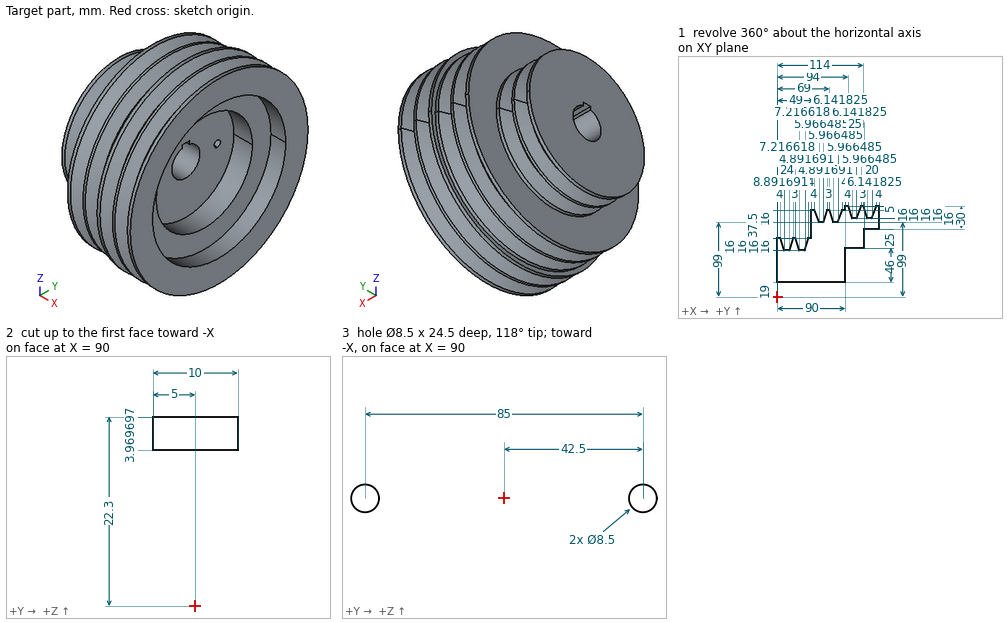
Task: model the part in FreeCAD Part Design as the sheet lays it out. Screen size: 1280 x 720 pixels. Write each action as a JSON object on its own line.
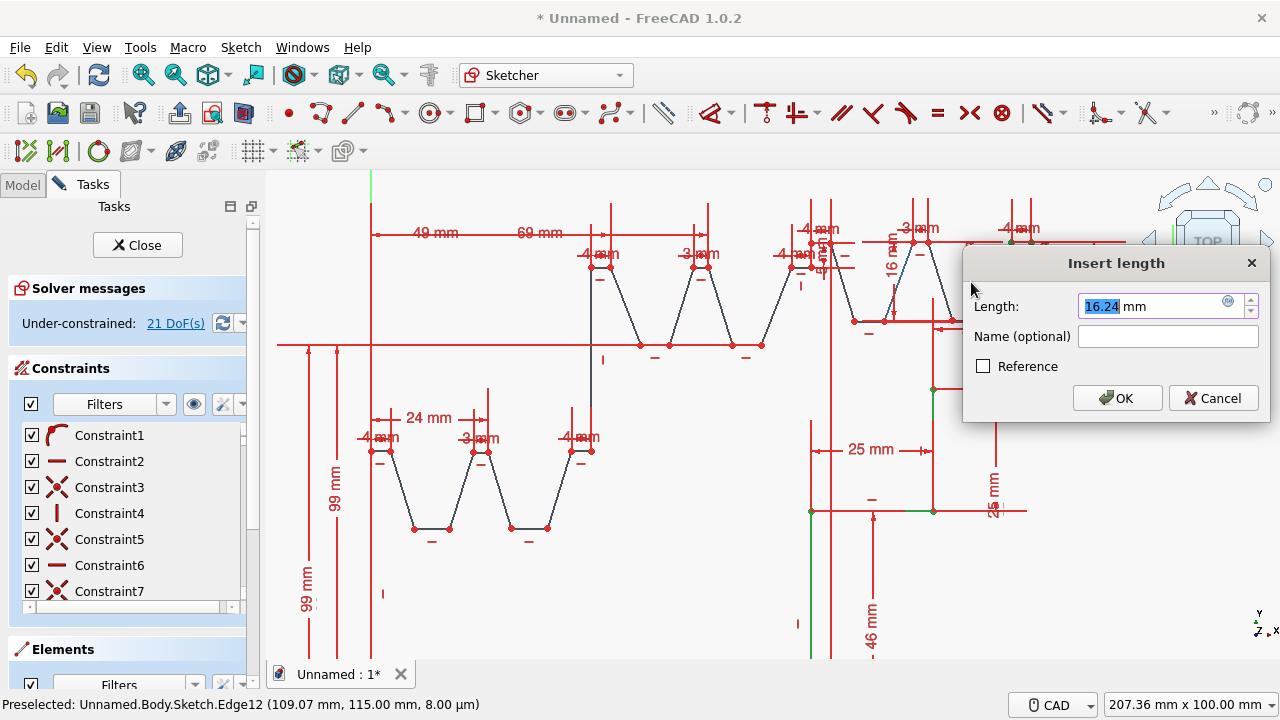
{"action": "type", "text": "16"}
{"action": "key", "text": "Return"}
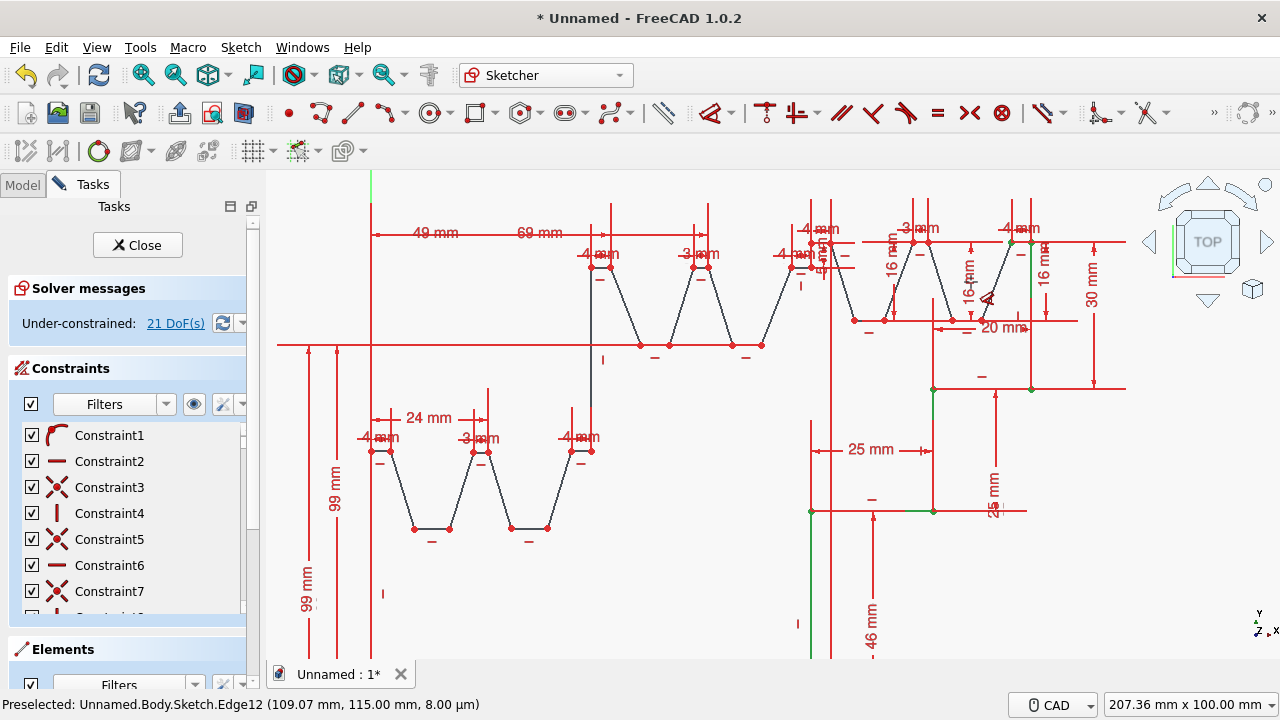
{"action": "left_click", "coordinate": [847, 297]}
{"action": "left_click", "coordinate": [797, 300]}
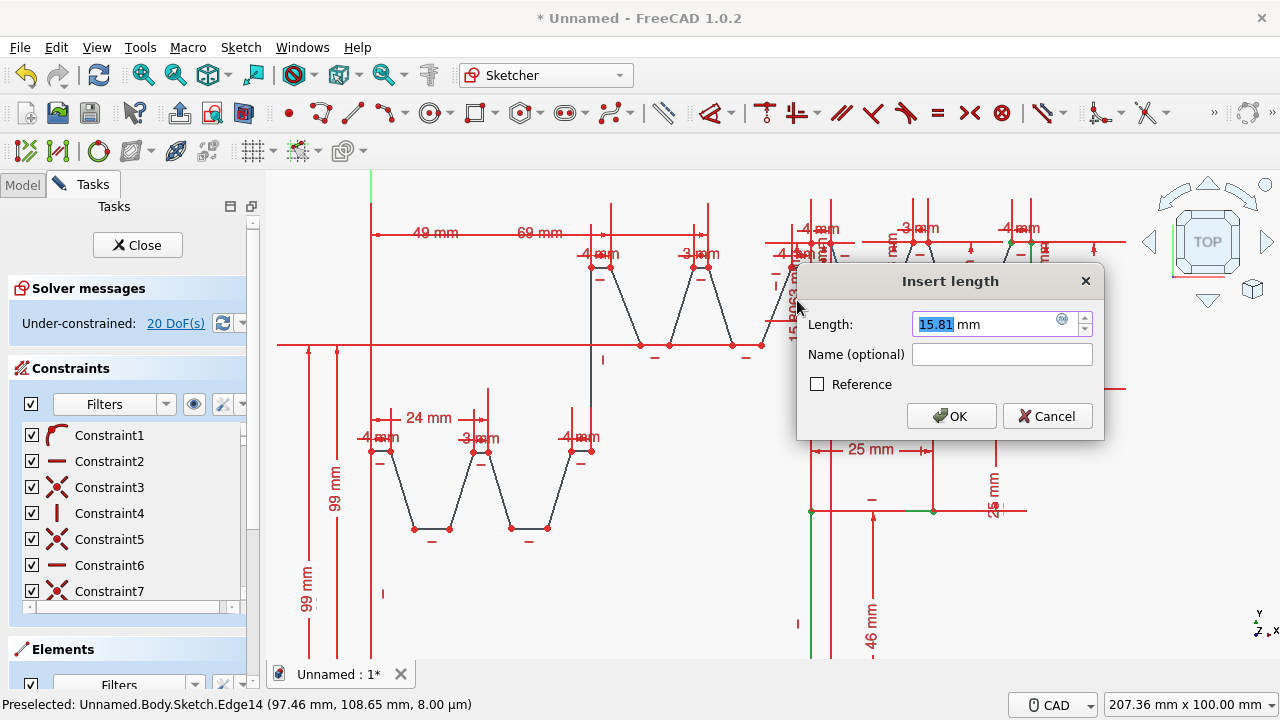
{"action": "type", "text": "16"}
{"action": "key", "text": "Return"}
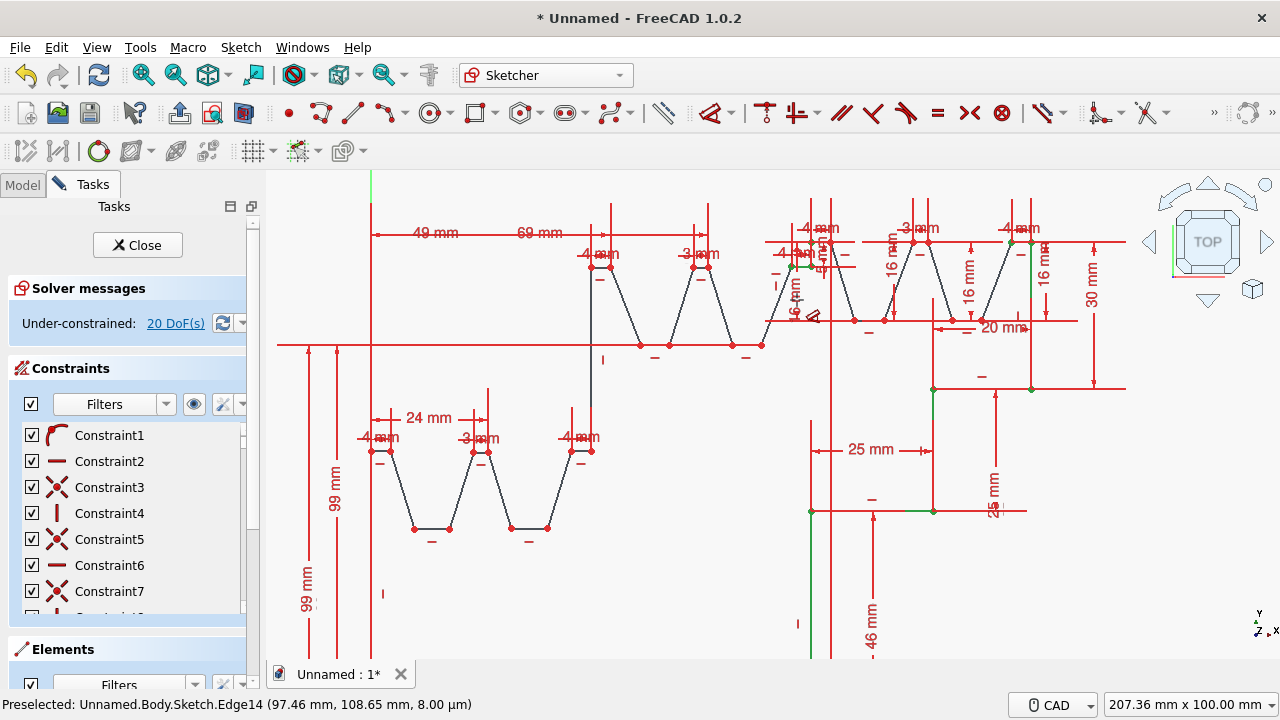
{"action": "left_click", "coordinate": [725, 322]}
{"action": "left_click", "coordinate": [767, 279]}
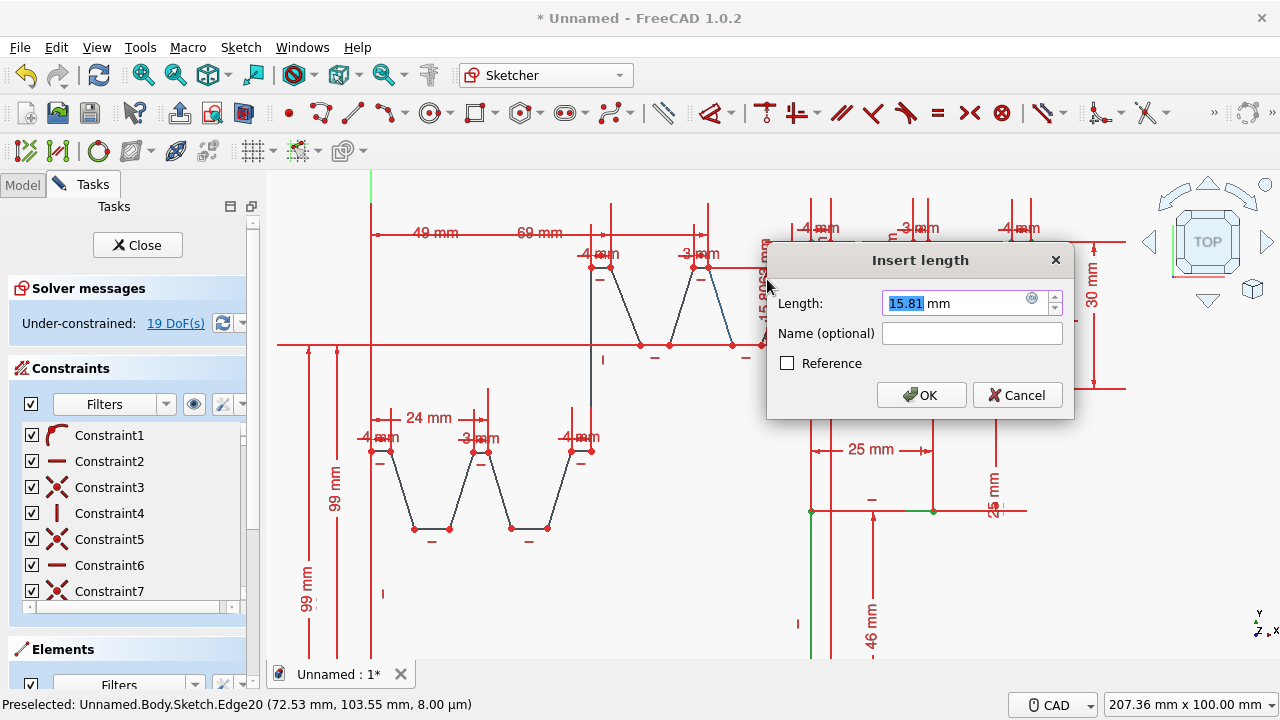
{"action": "type", "text": "16"}
{"action": "key", "text": "Return"}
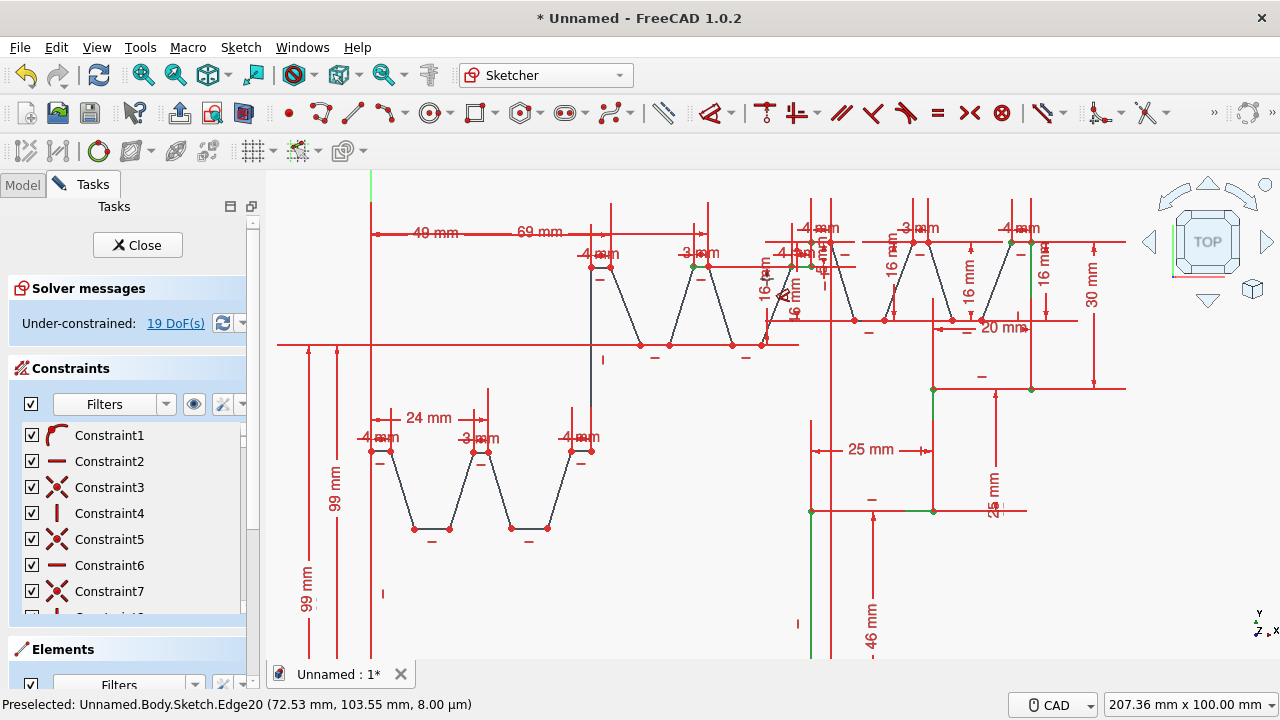
{"action": "left_click", "coordinate": [632, 322]}
{"action": "left_click", "coordinate": [577, 306]}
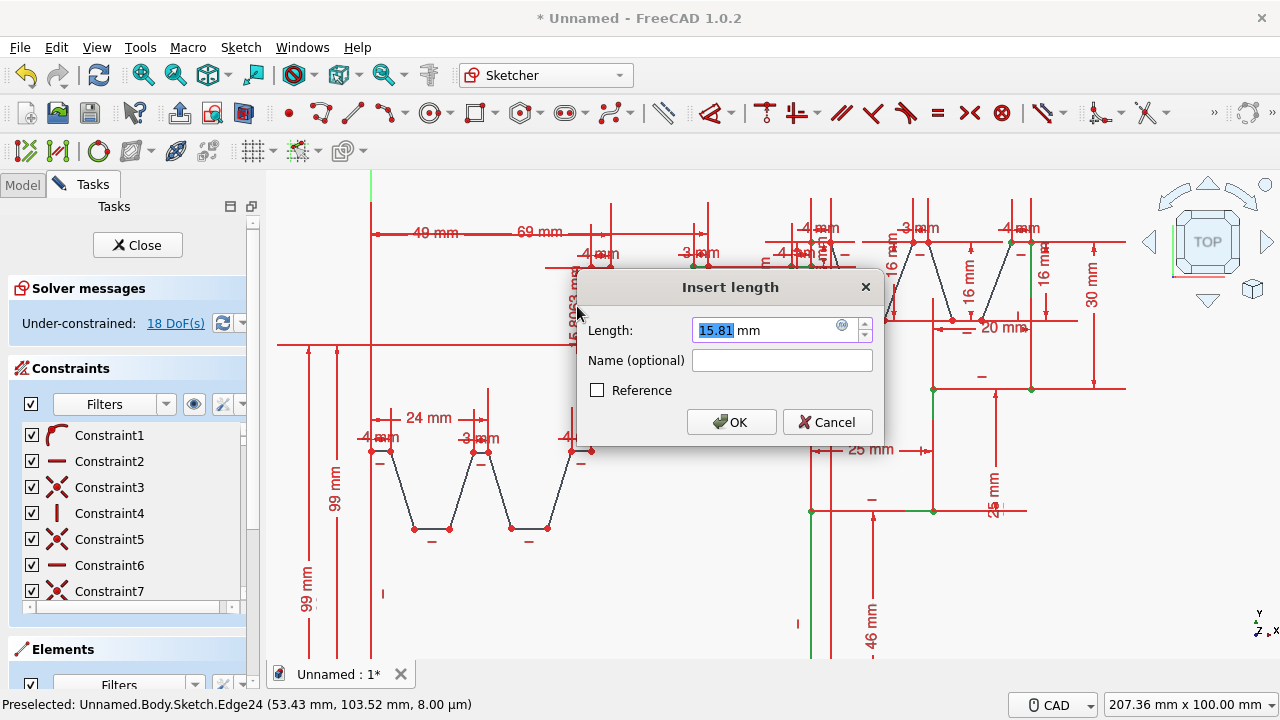
{"action": "type", "text": "16"}
{"action": "key", "text": "Return"}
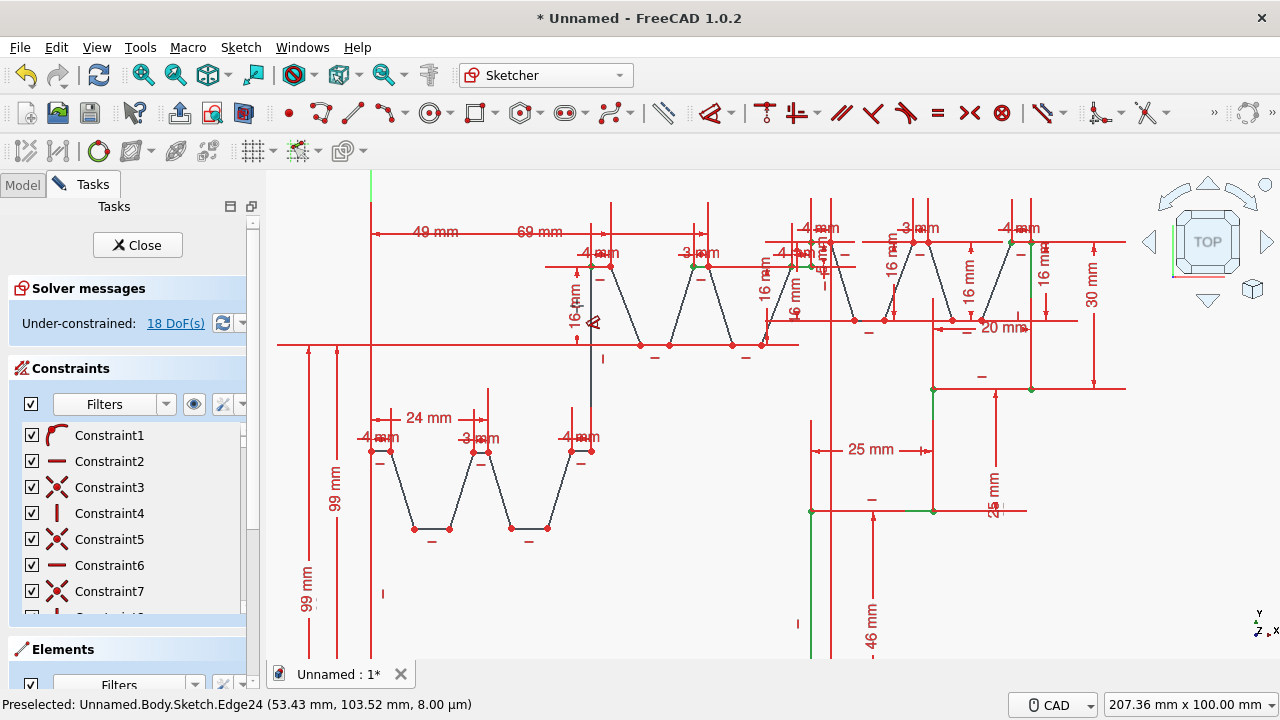
{"action": "left_click", "coordinate": [564, 474]}
{"action": "left_click", "coordinate": [514, 490]}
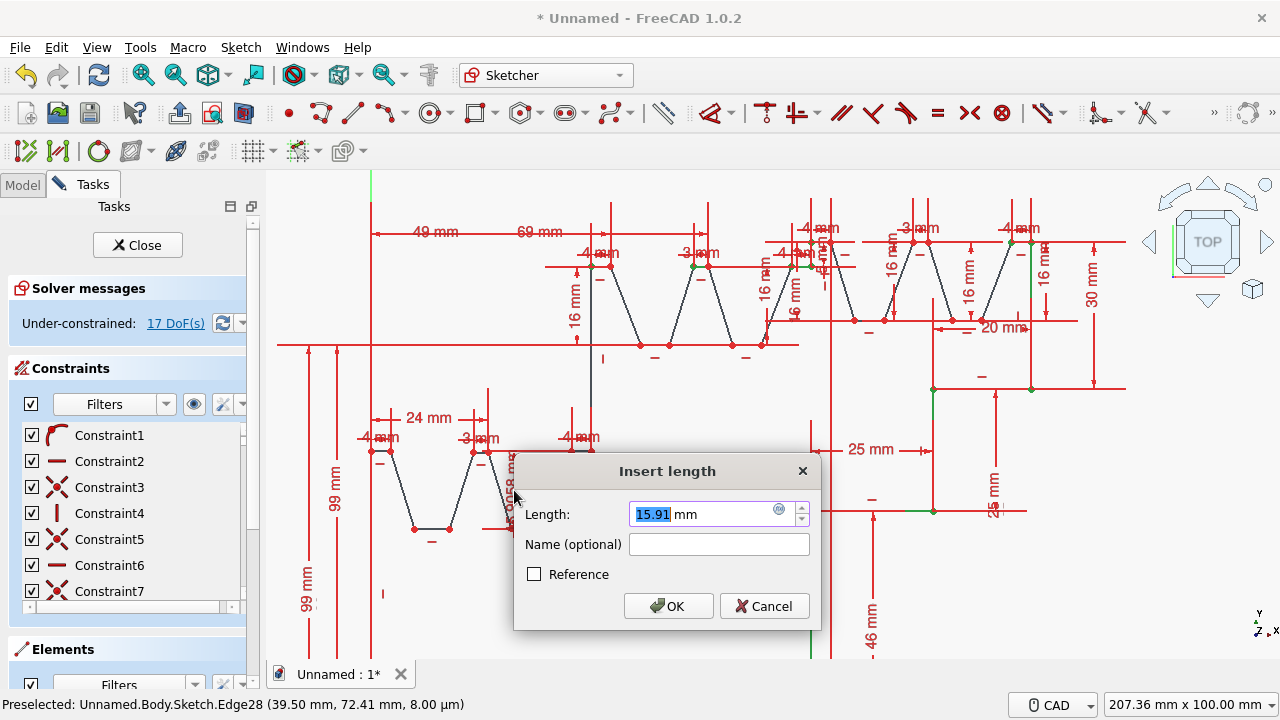
{"action": "type", "text": "16"}
{"action": "key", "text": "Return"}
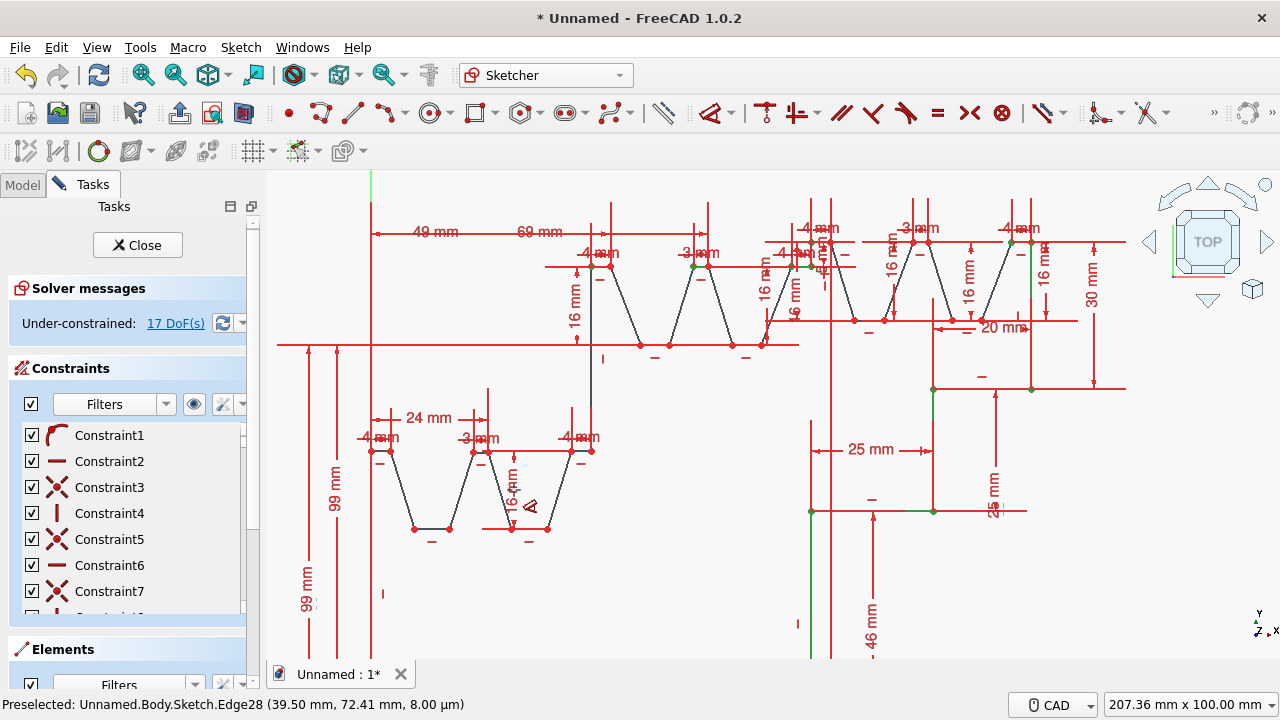
{"action": "left_click", "coordinate": [505, 506]}
{"action": "left_click", "coordinate": [454, 464]}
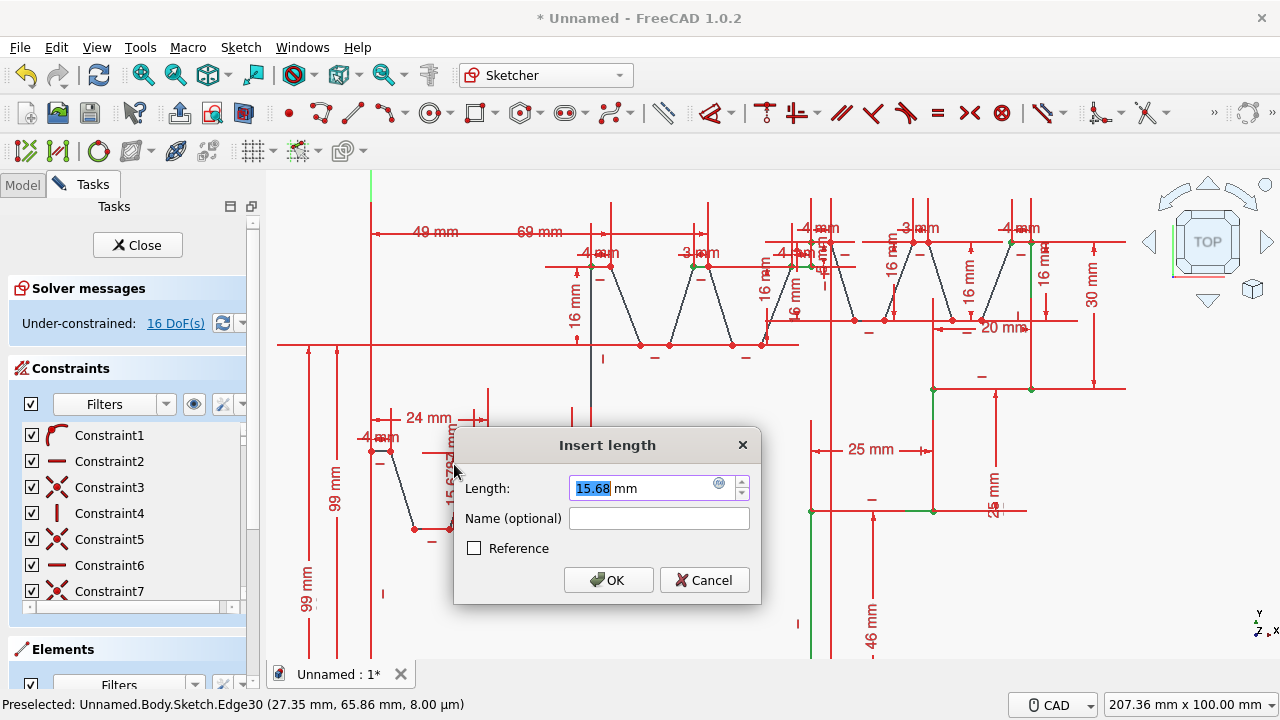
{"action": "type", "text": "16"}
{"action": "key", "text": "Return"}